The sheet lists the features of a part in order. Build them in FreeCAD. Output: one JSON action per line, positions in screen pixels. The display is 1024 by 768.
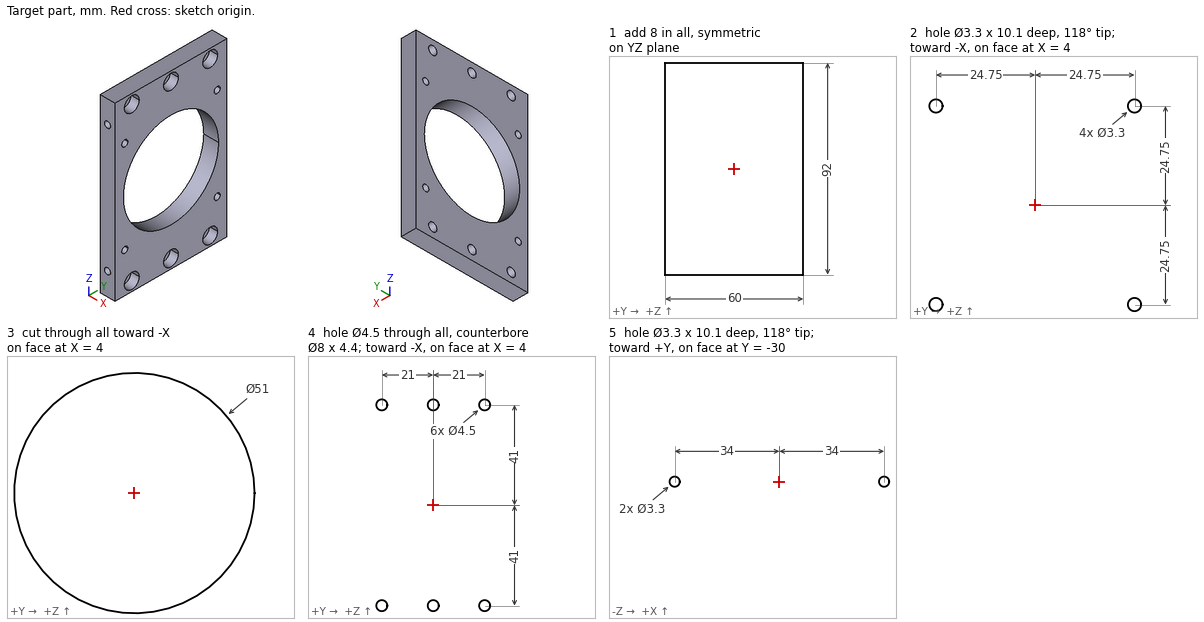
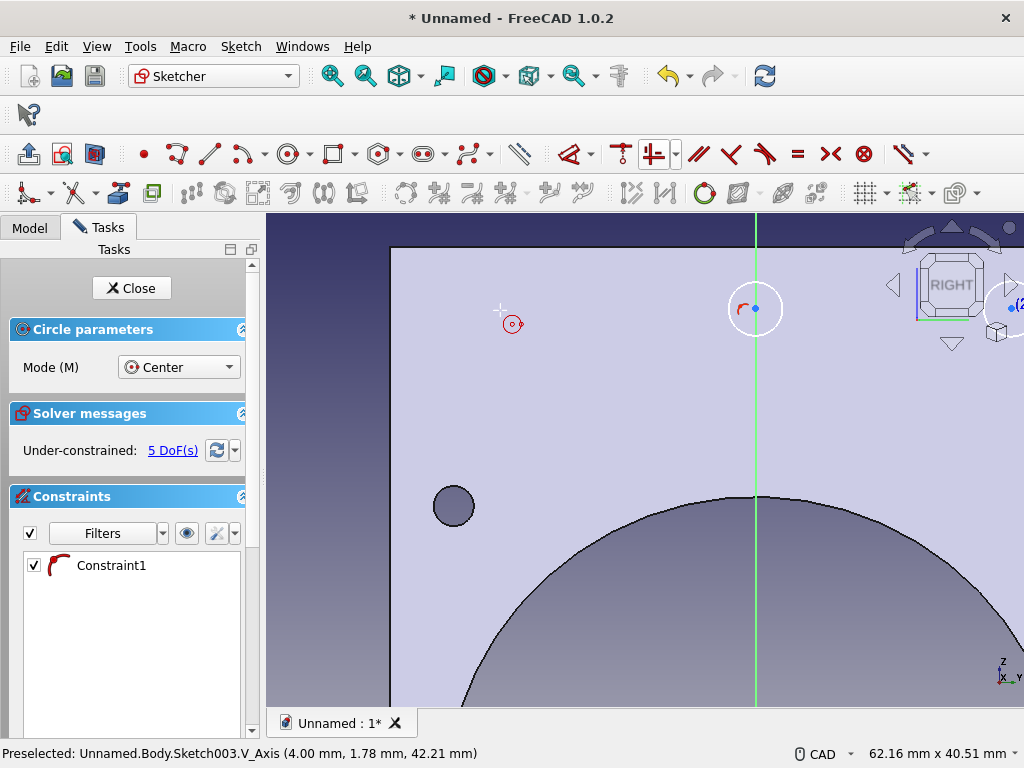
{"action": "left_click", "coordinate": [499, 308]}
{"action": "left_click", "coordinate": [519, 289]}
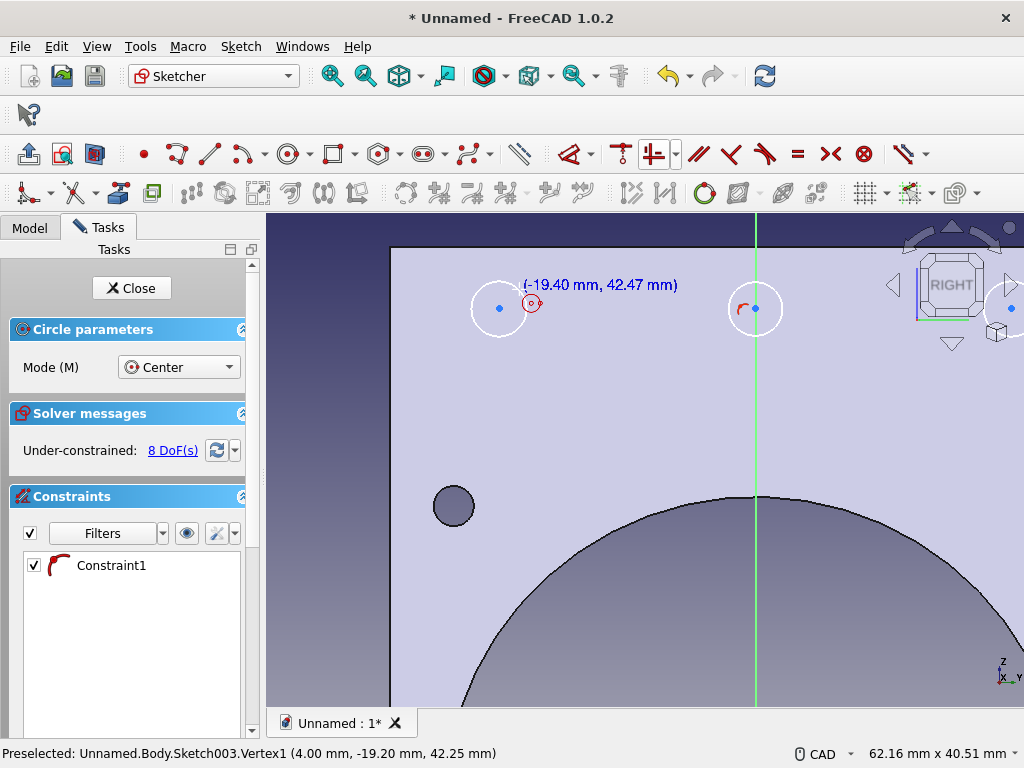
{"action": "scroll", "coordinate": [499, 310], "scroll_direction": "down", "scroll_amount": 6}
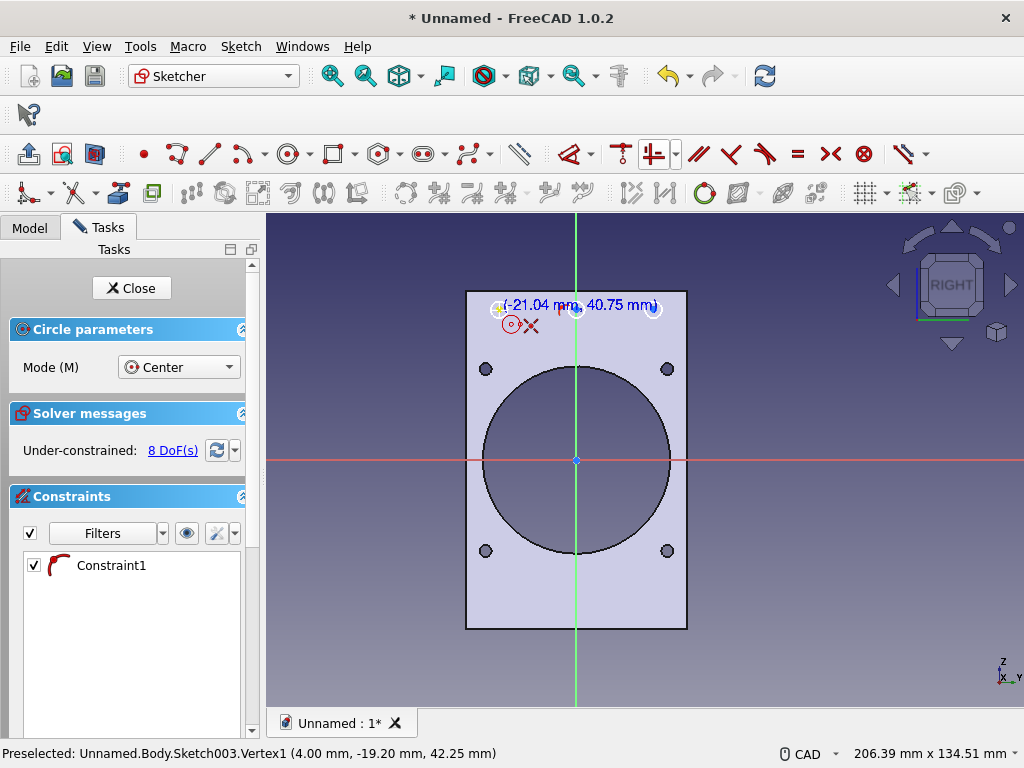
{"action": "scroll", "coordinate": [654, 611], "scroll_direction": "up", "scroll_amount": 6}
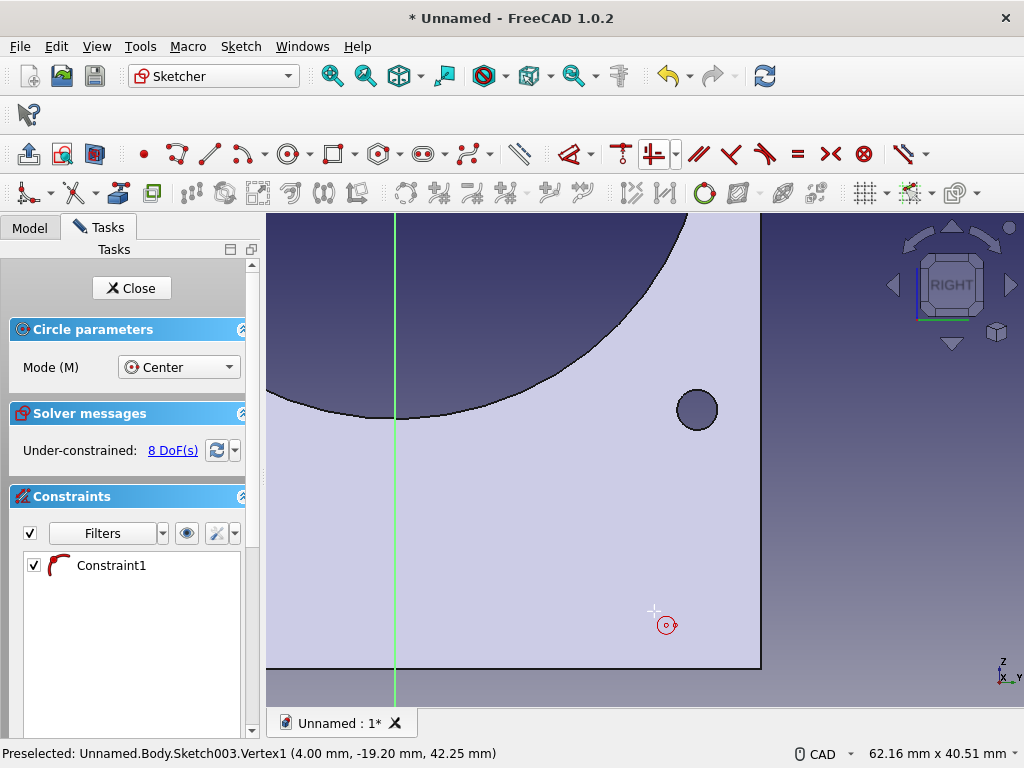
{"action": "left_click", "coordinate": [652, 608]}
{"action": "left_click", "coordinate": [671, 589]}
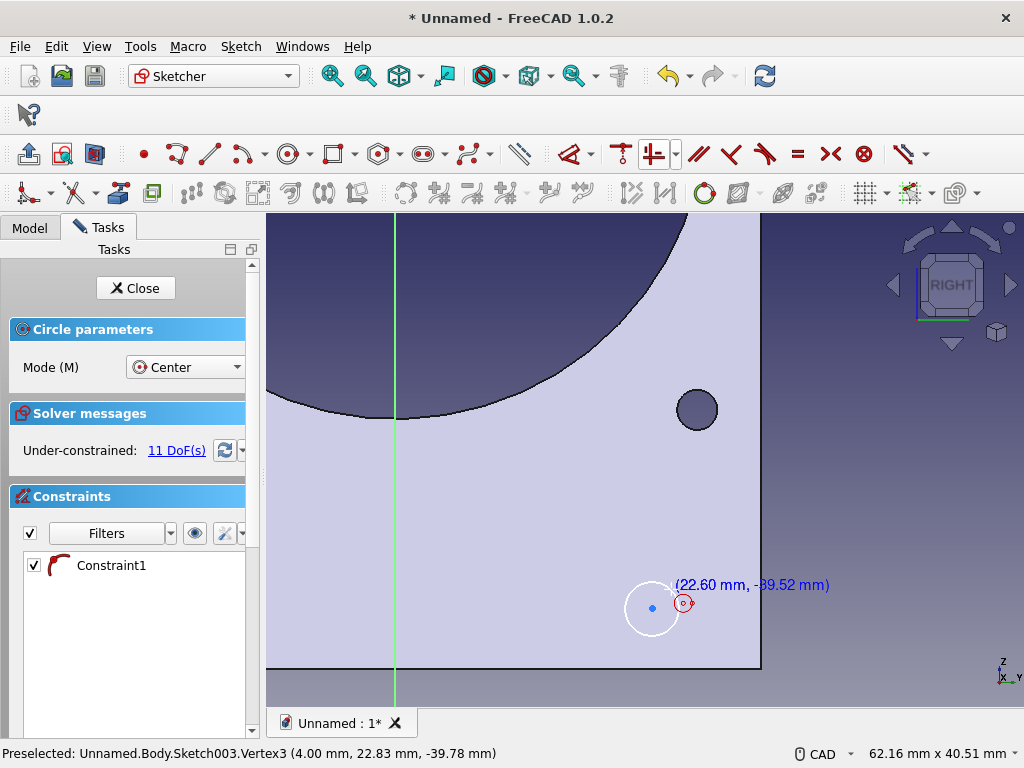
{"action": "left_click", "coordinate": [395, 608]}
{"action": "left_click", "coordinate": [415, 589]}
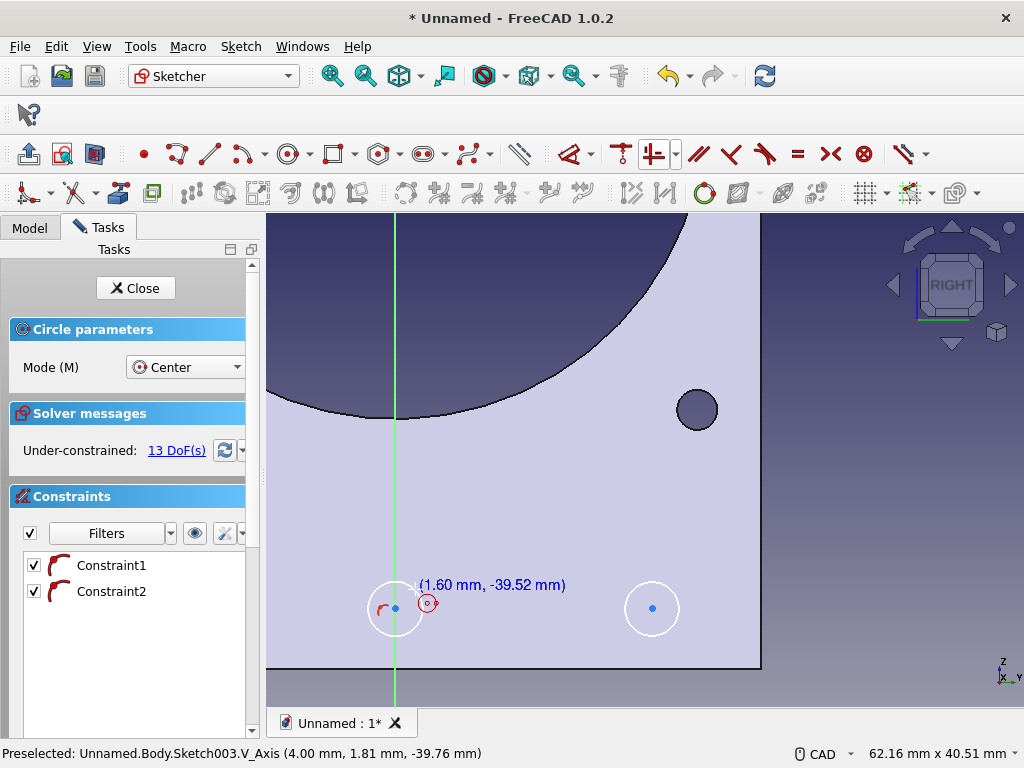
{"action": "scroll", "coordinate": [655, 612], "scroll_direction": "down", "scroll_amount": 6}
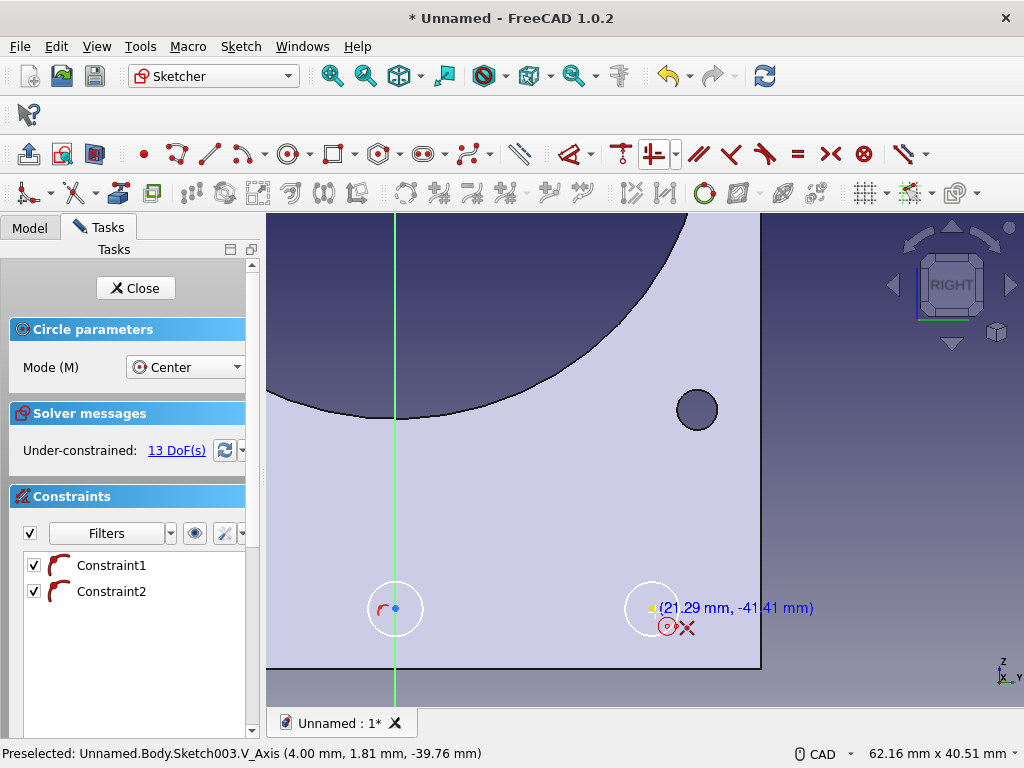
{"action": "scroll", "coordinate": [500, 611], "scroll_direction": "up", "scroll_amount": 6}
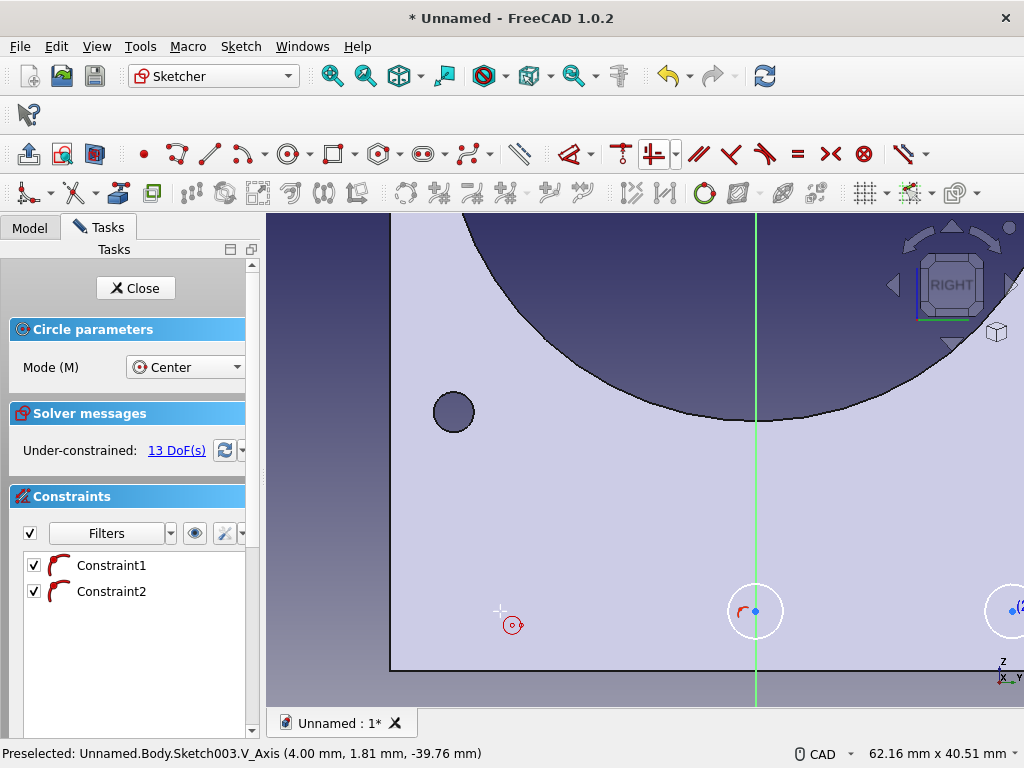
{"action": "left_click", "coordinate": [499, 610]}
{"action": "left_click", "coordinate": [519, 591]}
{"action": "key", "text": "Escape"}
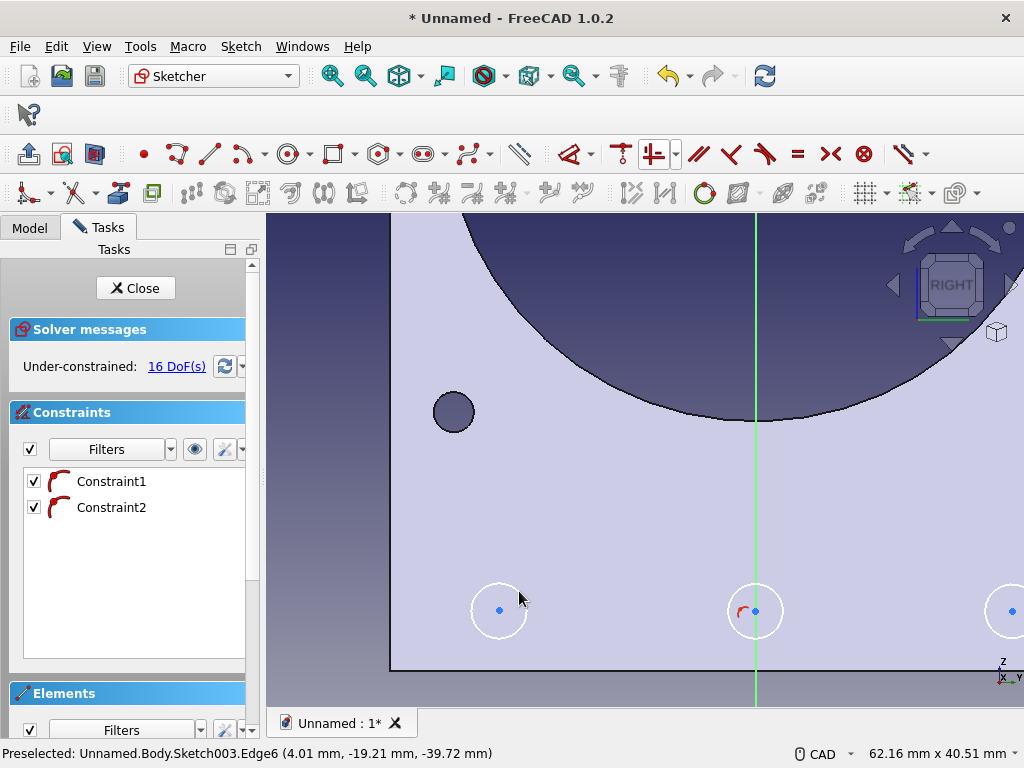
{"action": "scroll", "coordinate": [499, 611], "scroll_direction": "down", "scroll_amount": 6}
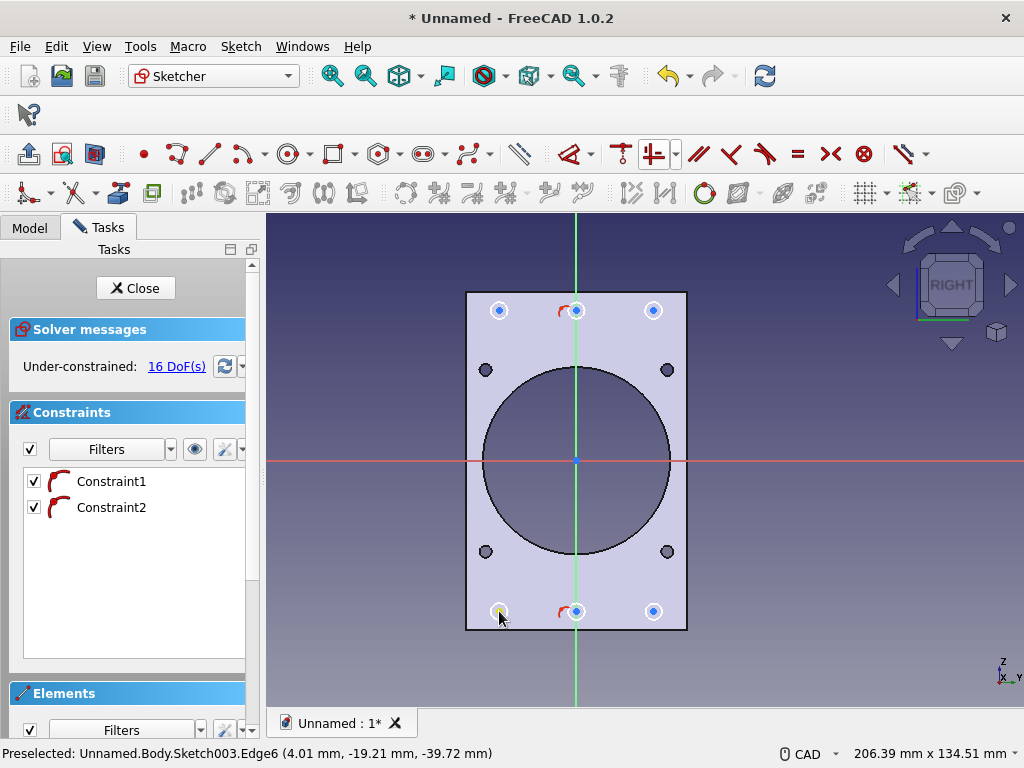
{"action": "scroll", "coordinate": [659, 305], "scroll_direction": "up", "scroll_amount": 3}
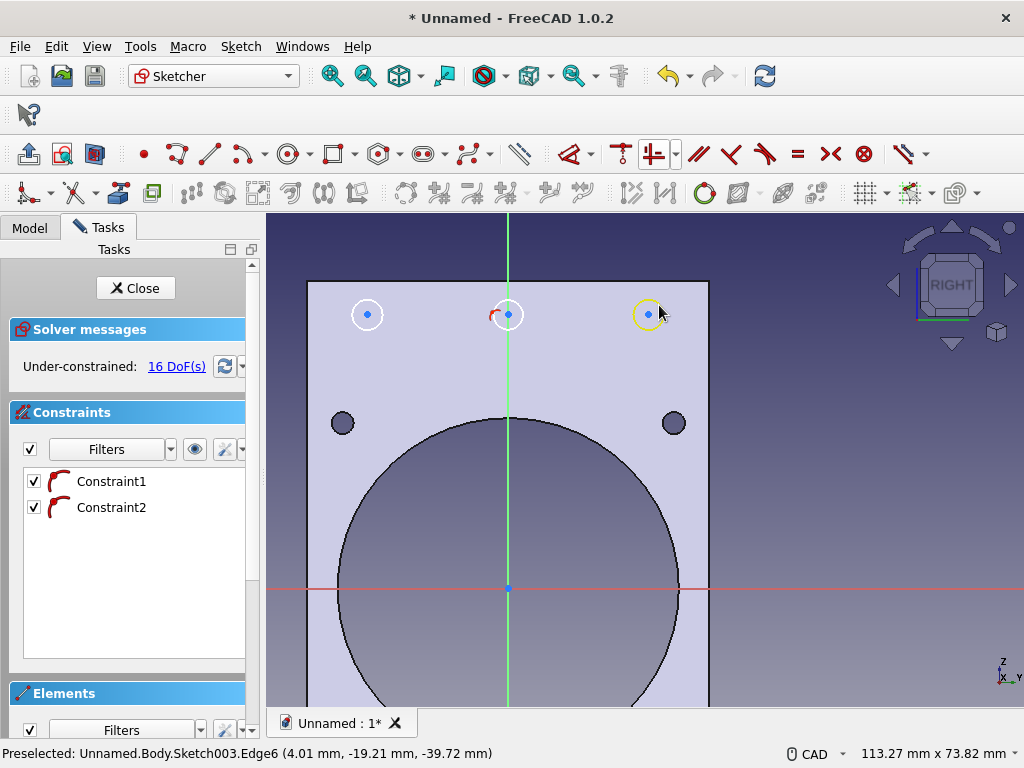
{"action": "left_click", "coordinate": [659, 304]}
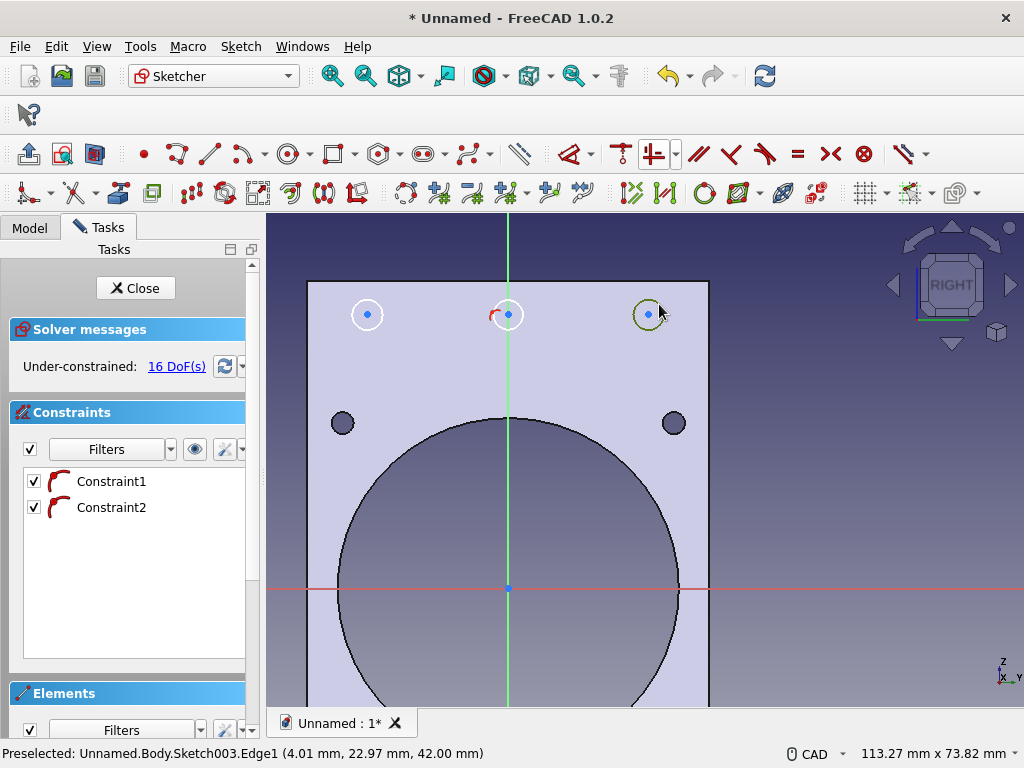
{"action": "scroll", "coordinate": [519, 305], "scroll_direction": "up", "scroll_amount": 2}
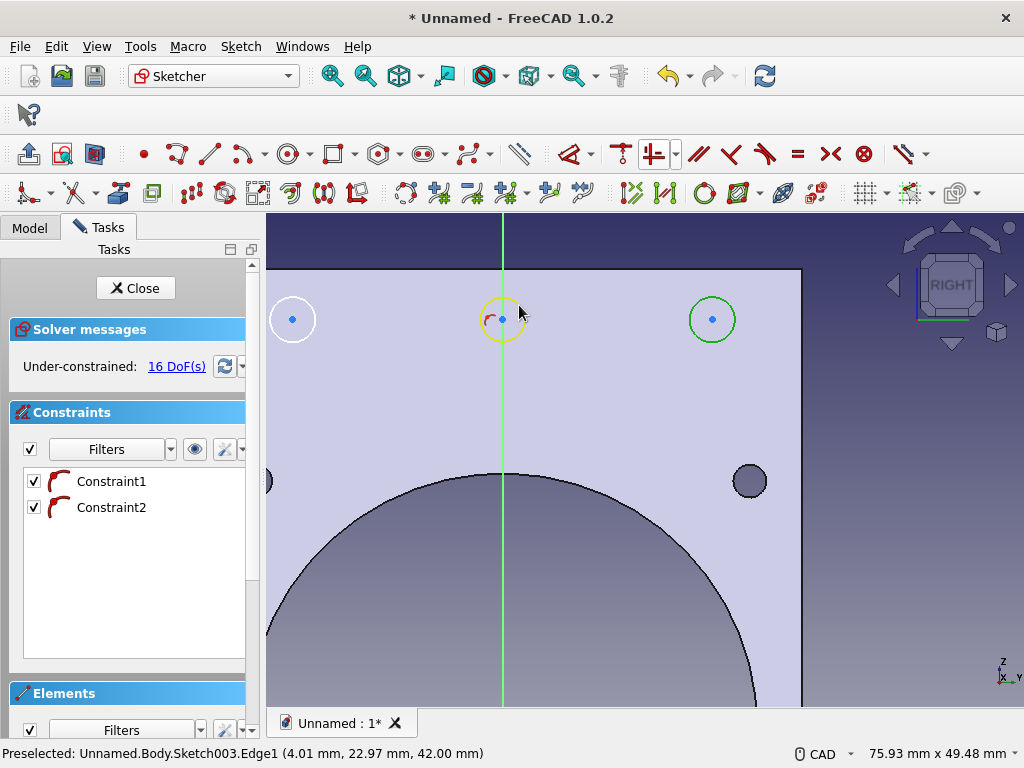
{"action": "left_click", "coordinate": [518, 304]}